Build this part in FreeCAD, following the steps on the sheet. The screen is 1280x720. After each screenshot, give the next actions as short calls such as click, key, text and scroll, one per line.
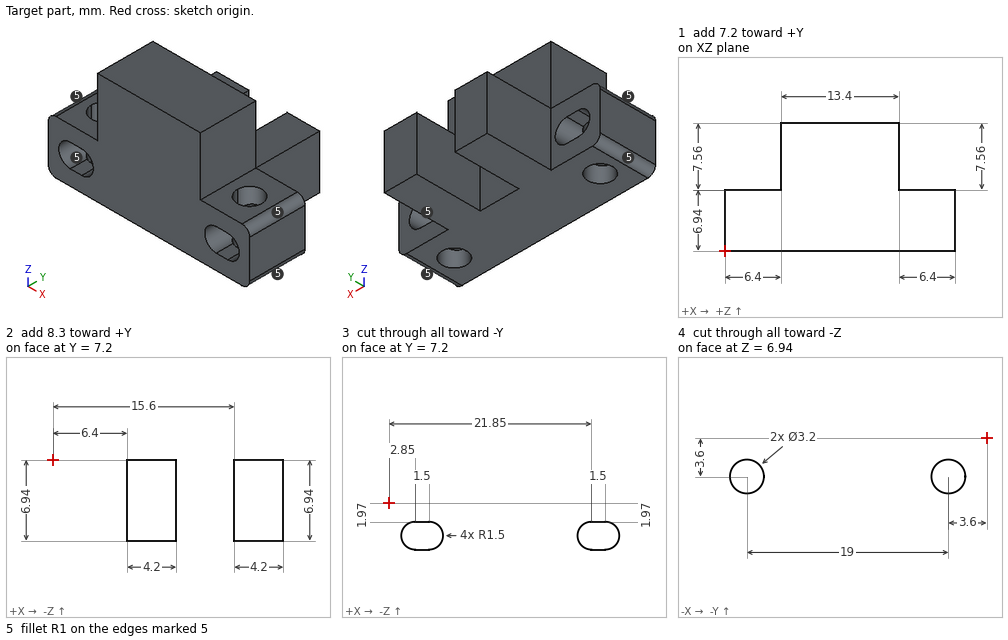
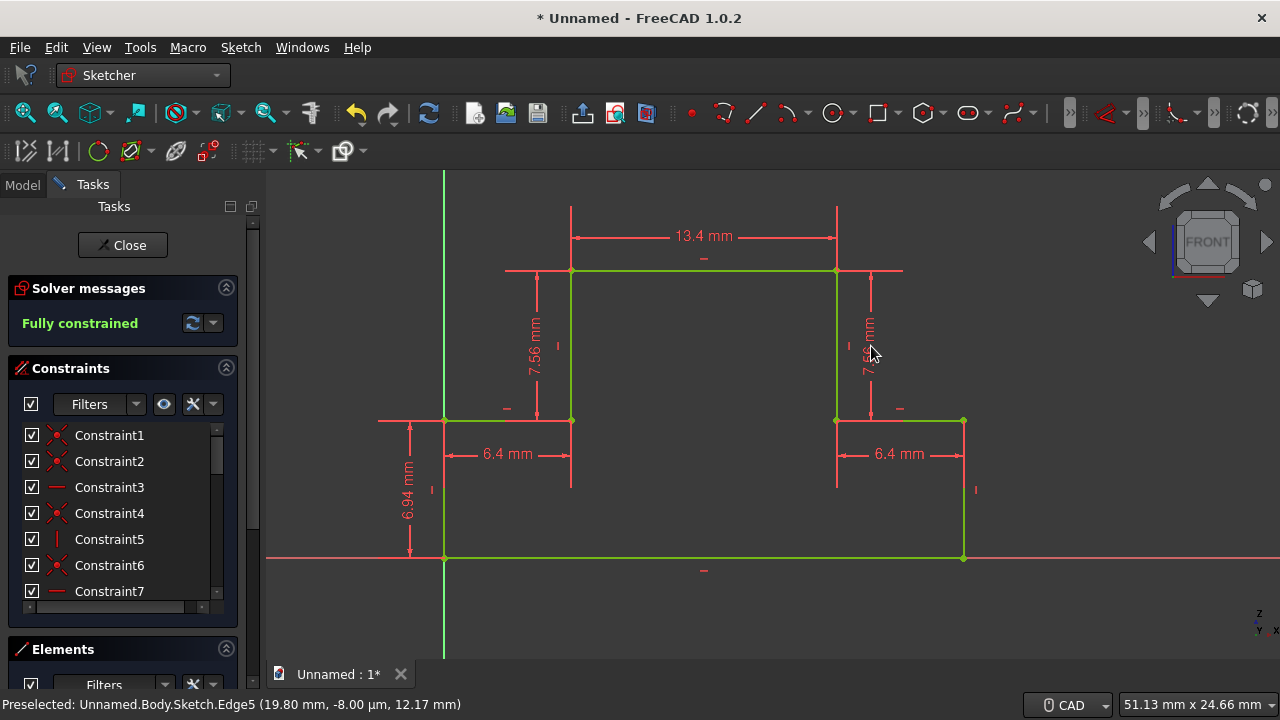
click(123, 245)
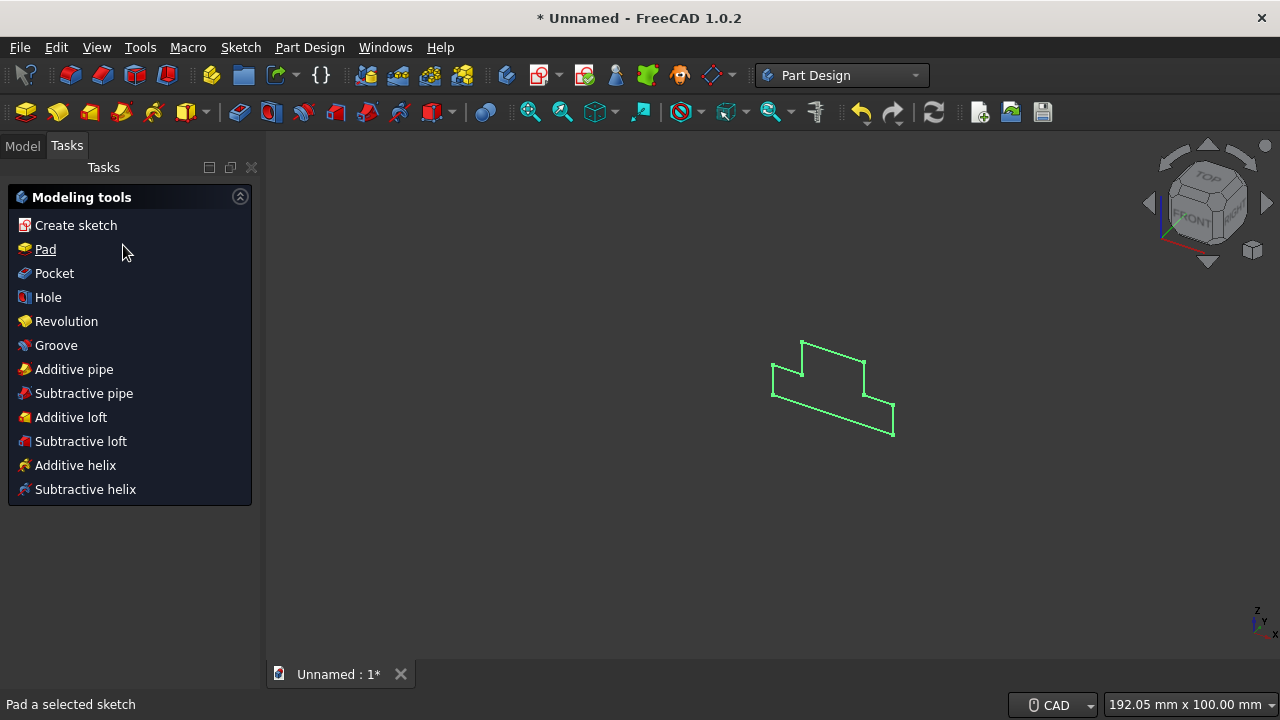
click(26, 112)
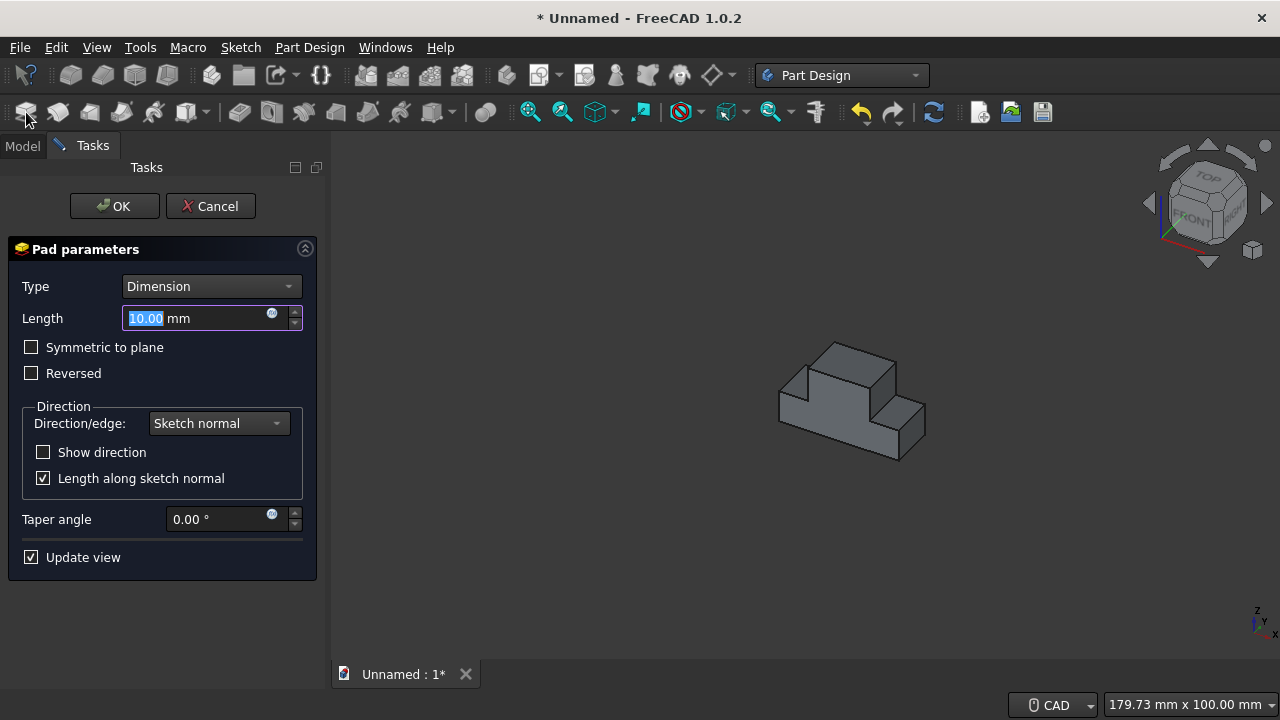
text(7.2)
key(Tab)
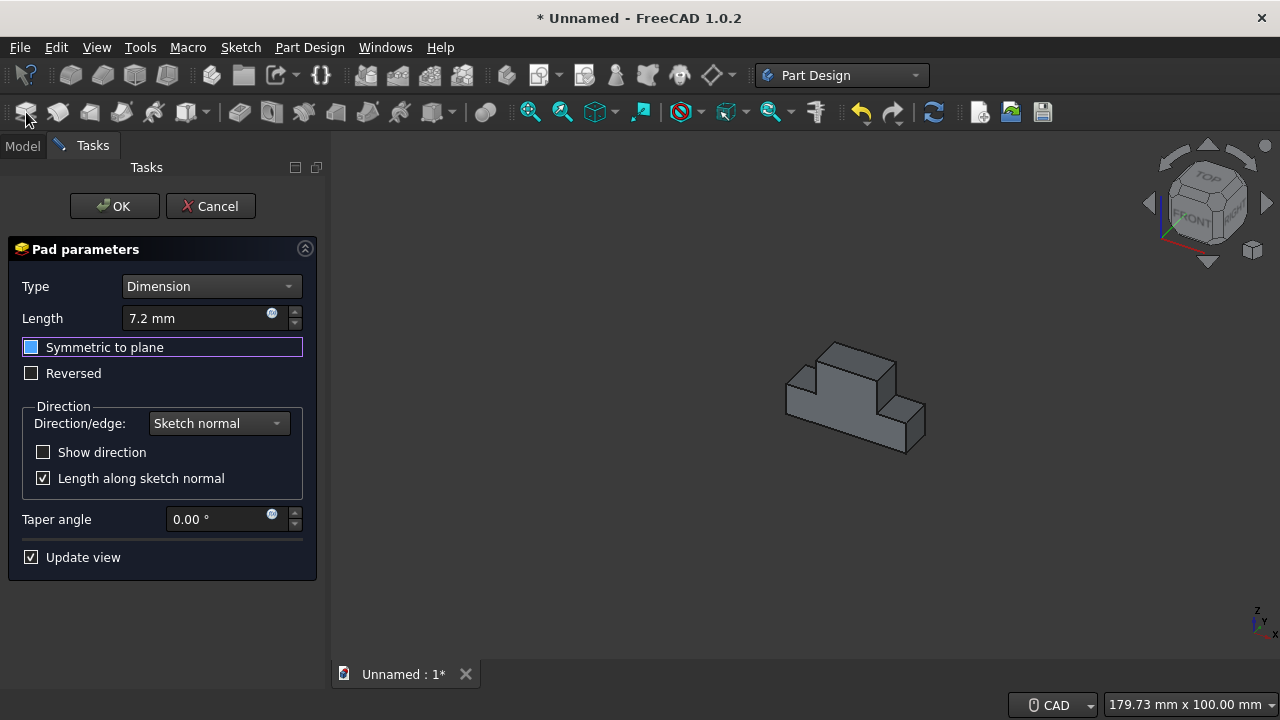
click(30, 373)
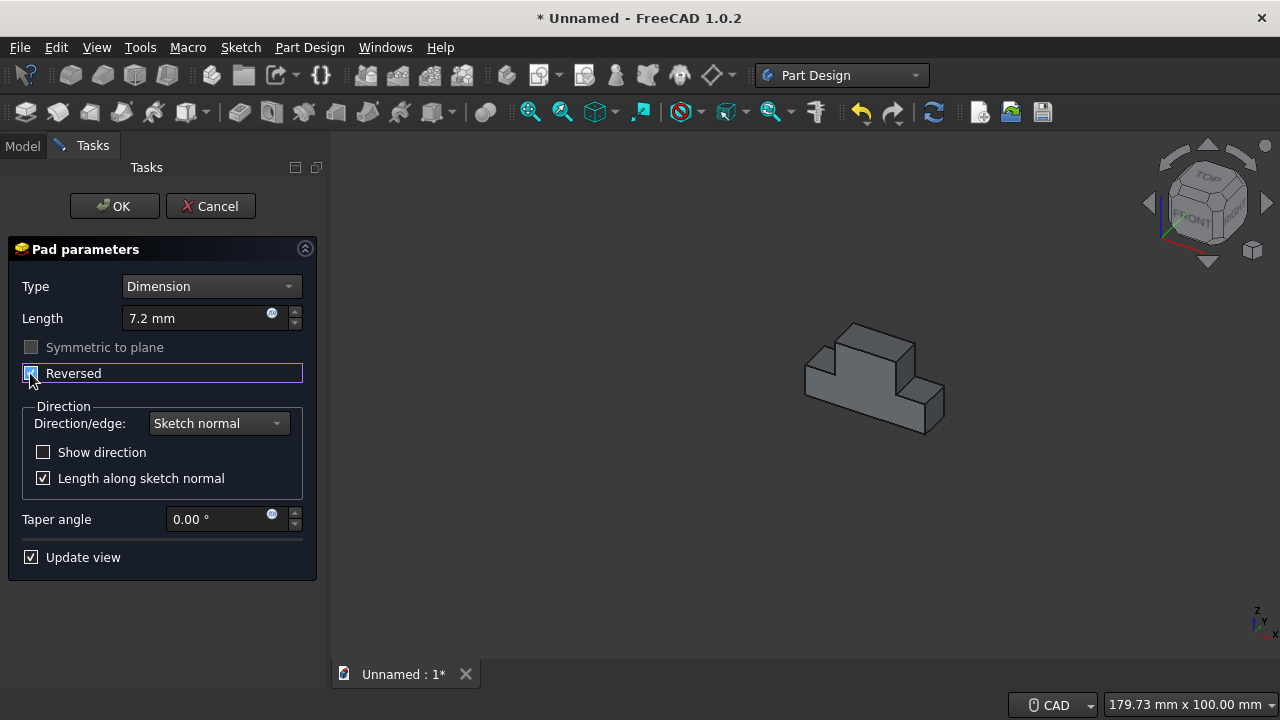
click(115, 206)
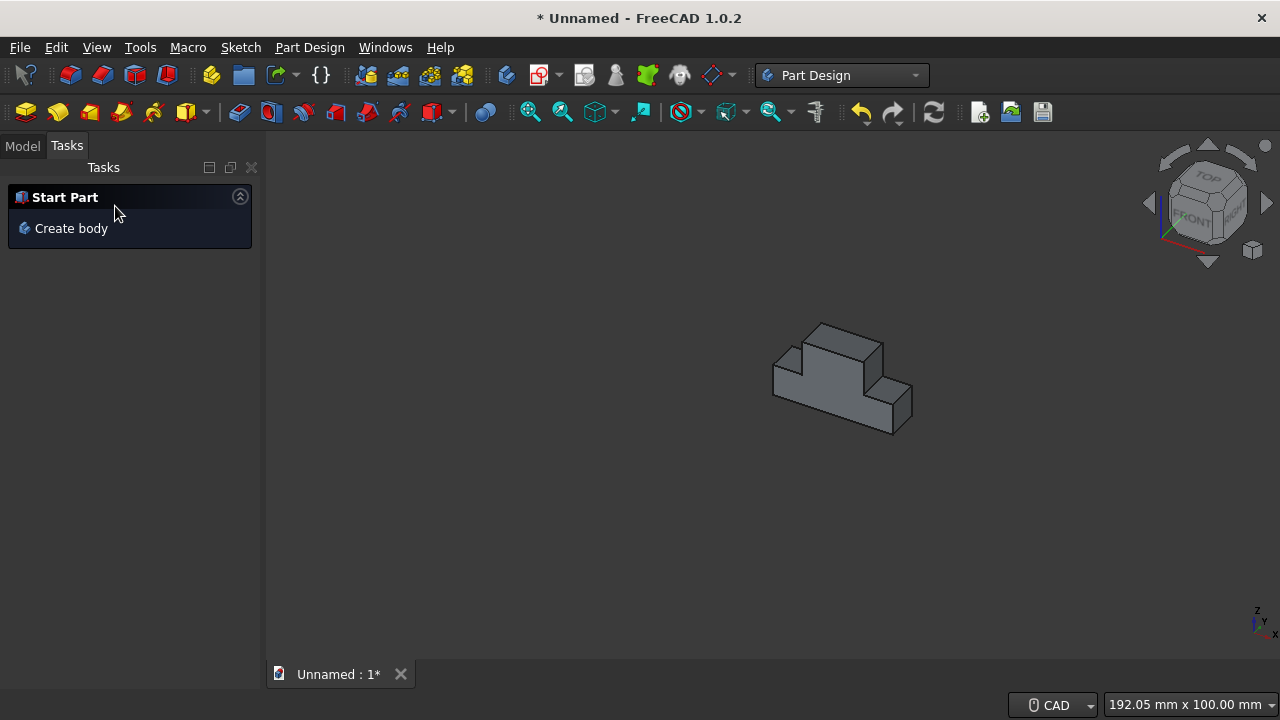
click(532, 112)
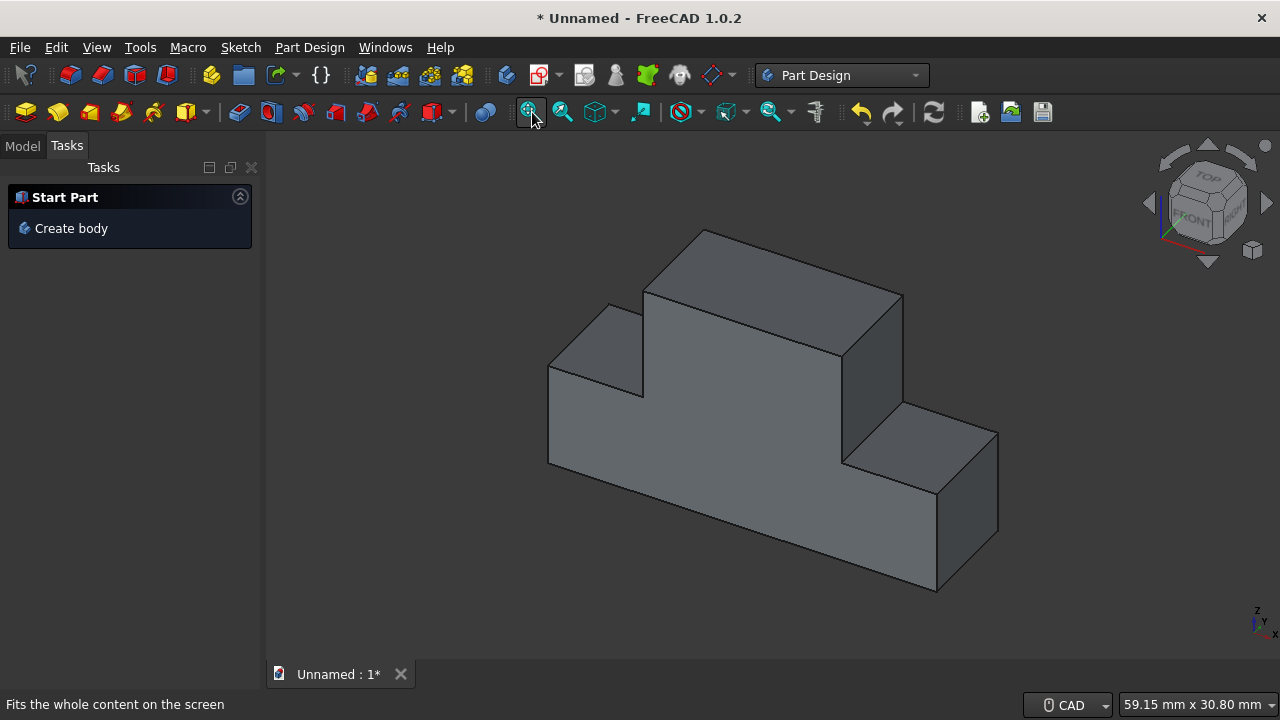
key(4)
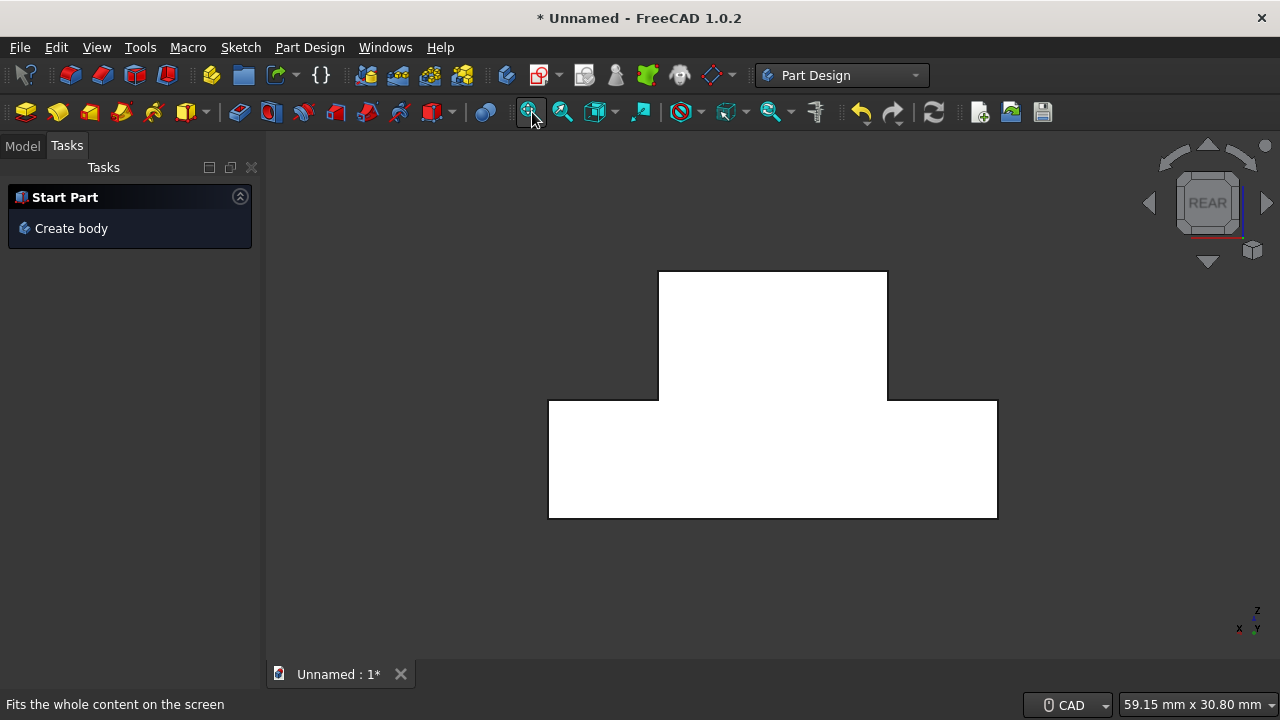
click(773, 394)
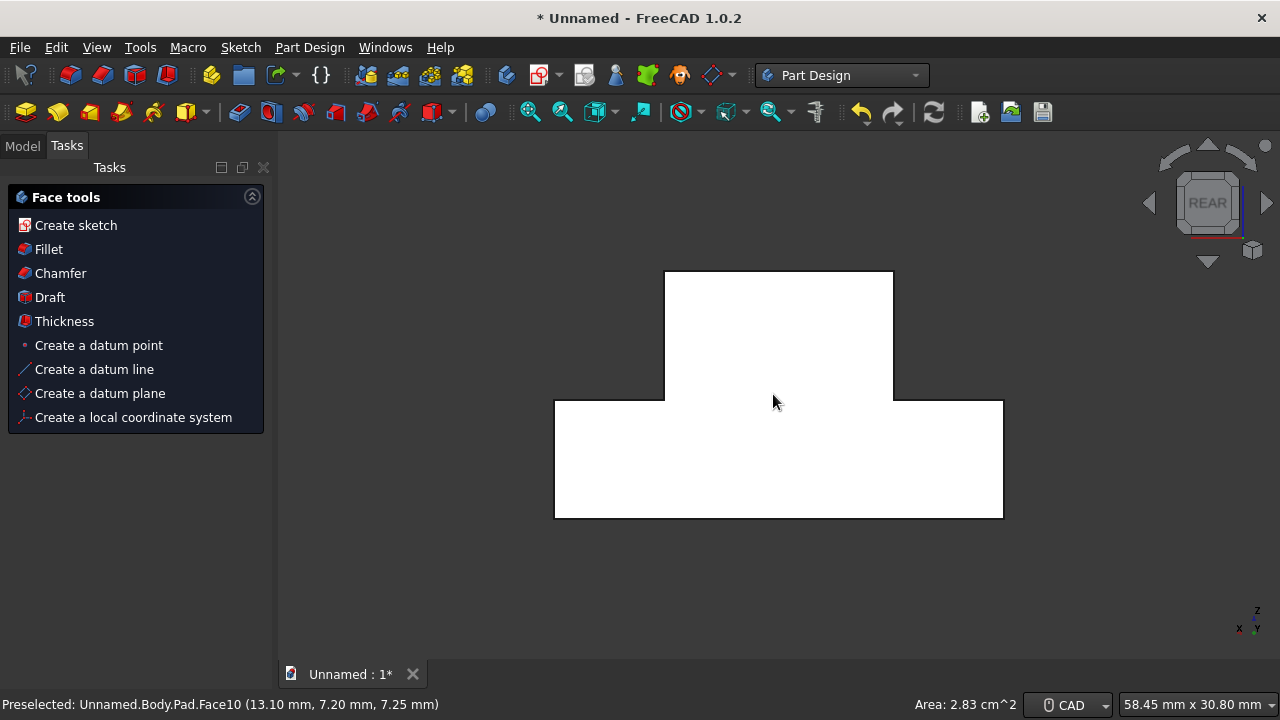
click(540, 76)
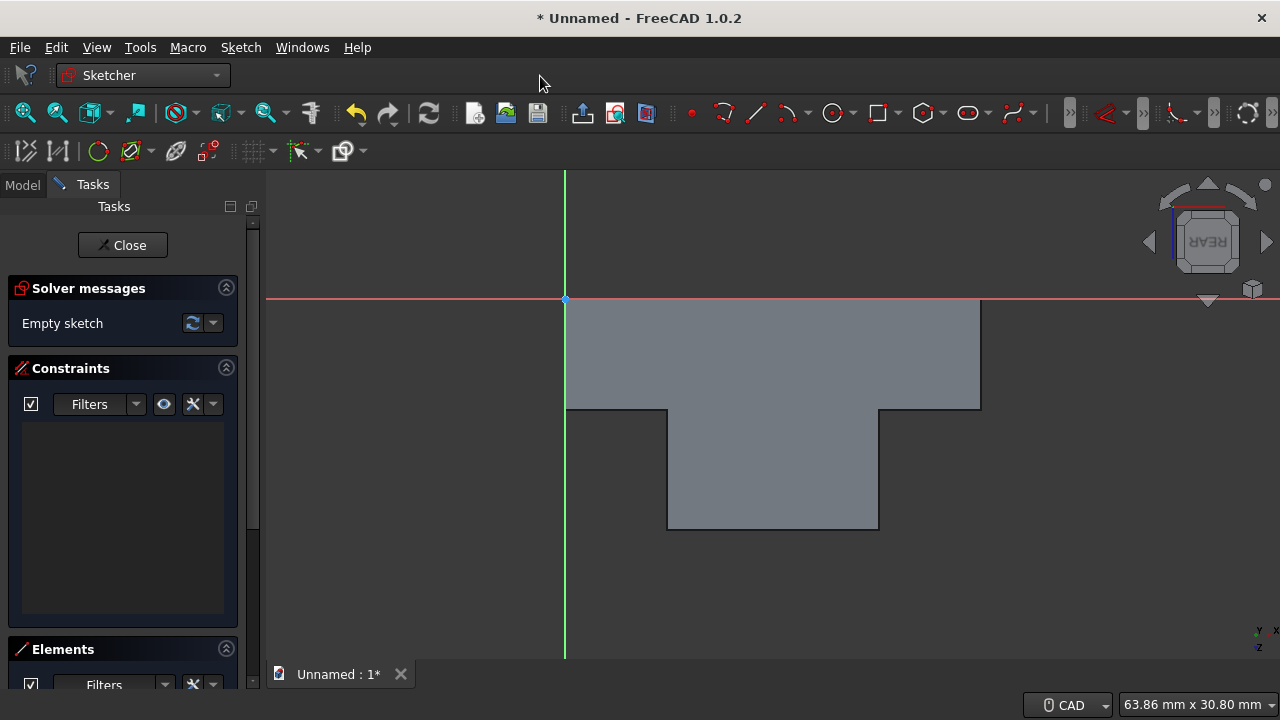
scroll(744, 281, up, 3)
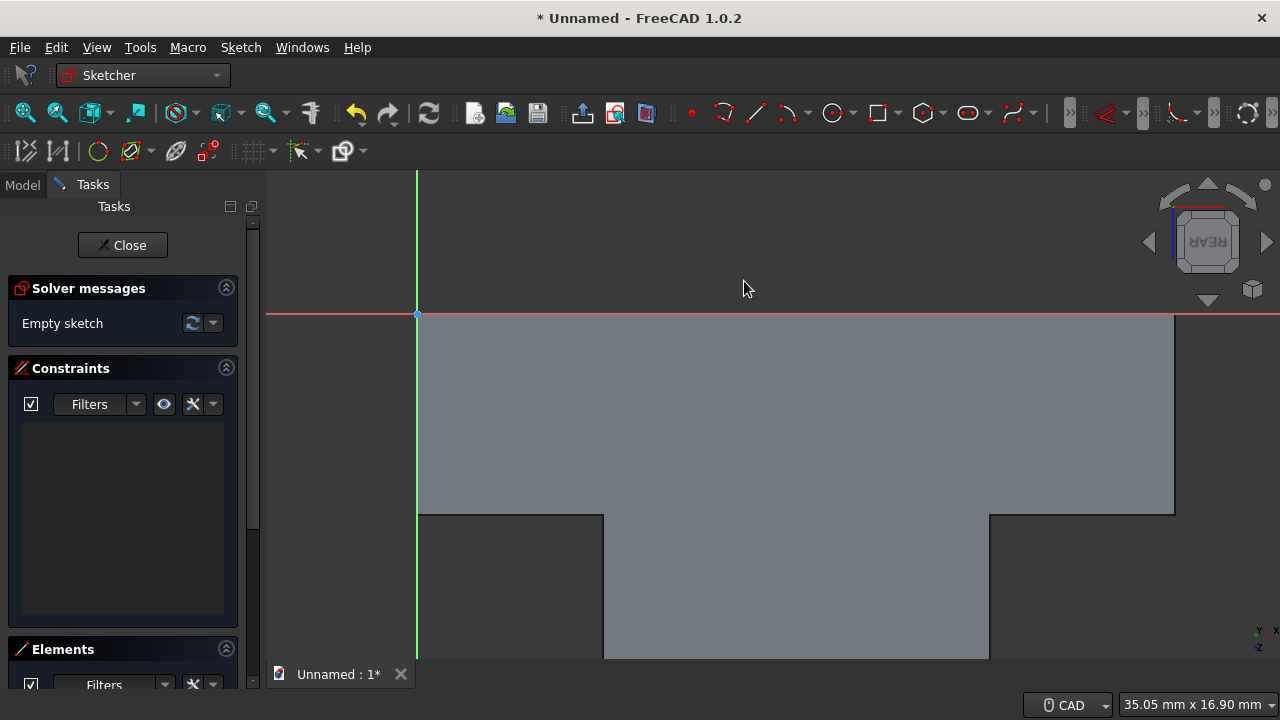
click(878, 114)